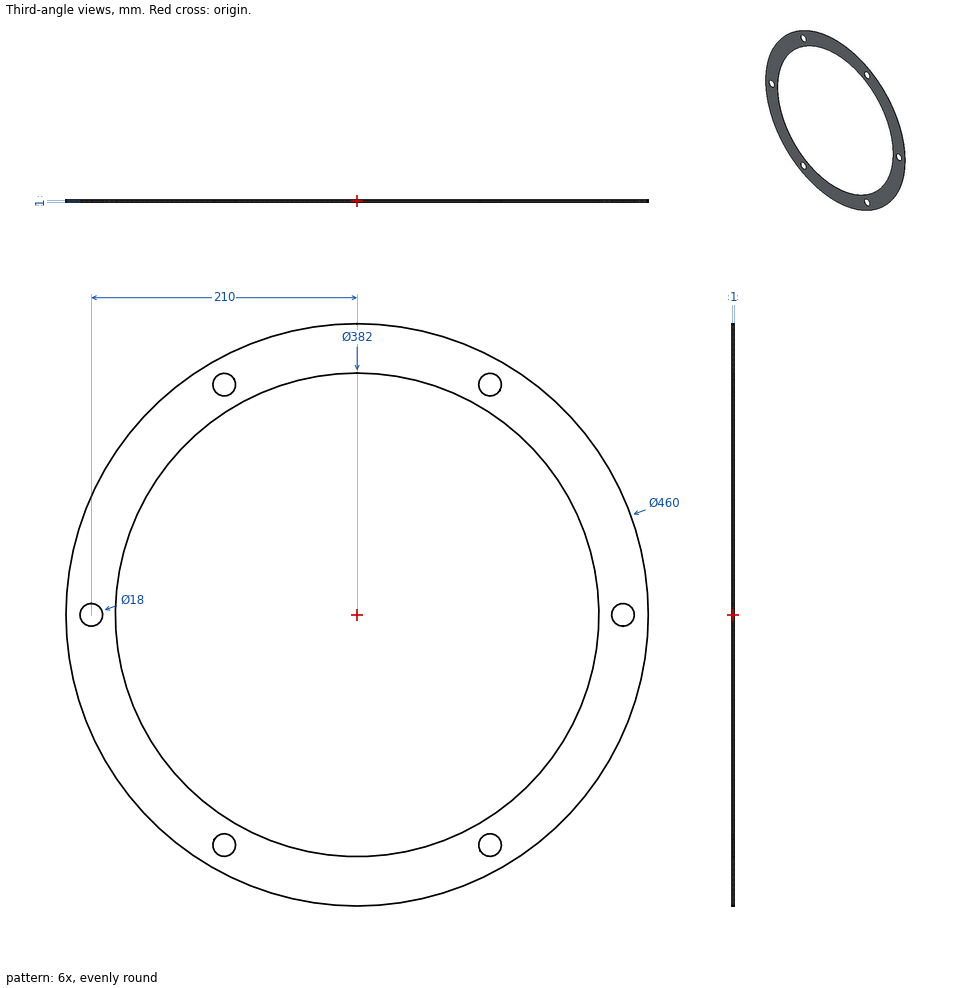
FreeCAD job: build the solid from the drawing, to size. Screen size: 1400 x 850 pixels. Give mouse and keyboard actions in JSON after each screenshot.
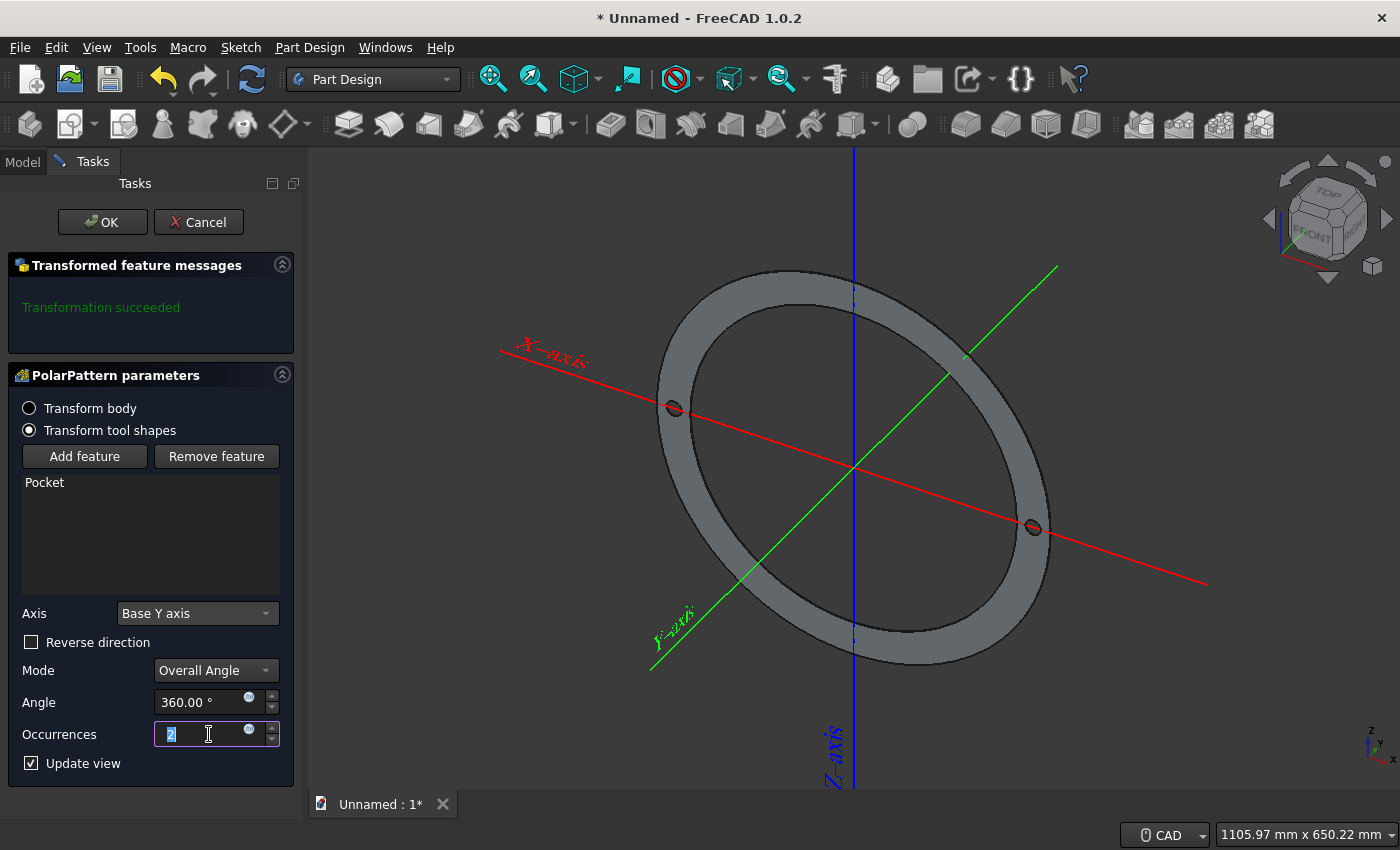
{"action": "type", "text": "6"}
{"action": "key", "text": "Tab"}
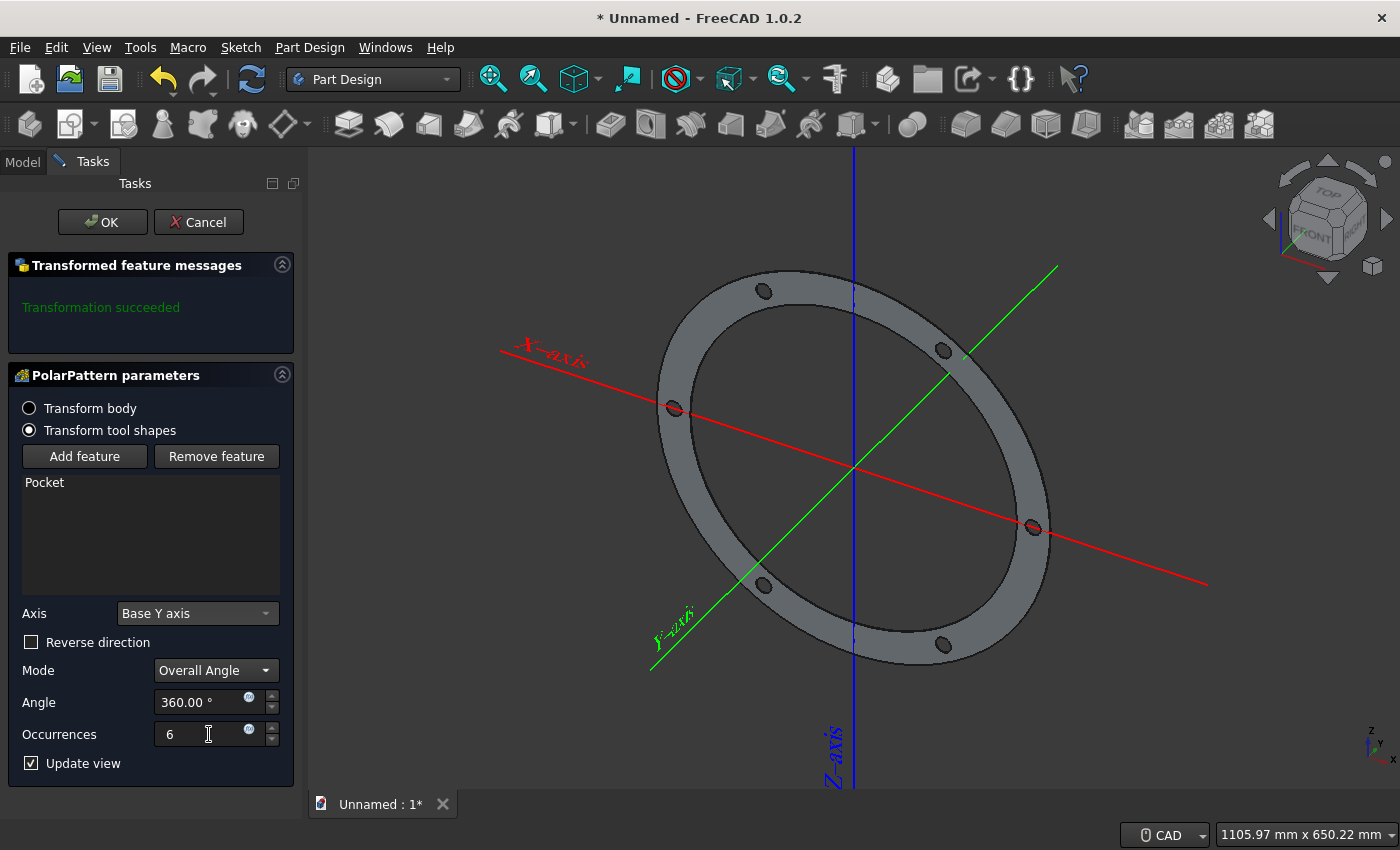
{"action": "left_click", "coordinate": [103, 222]}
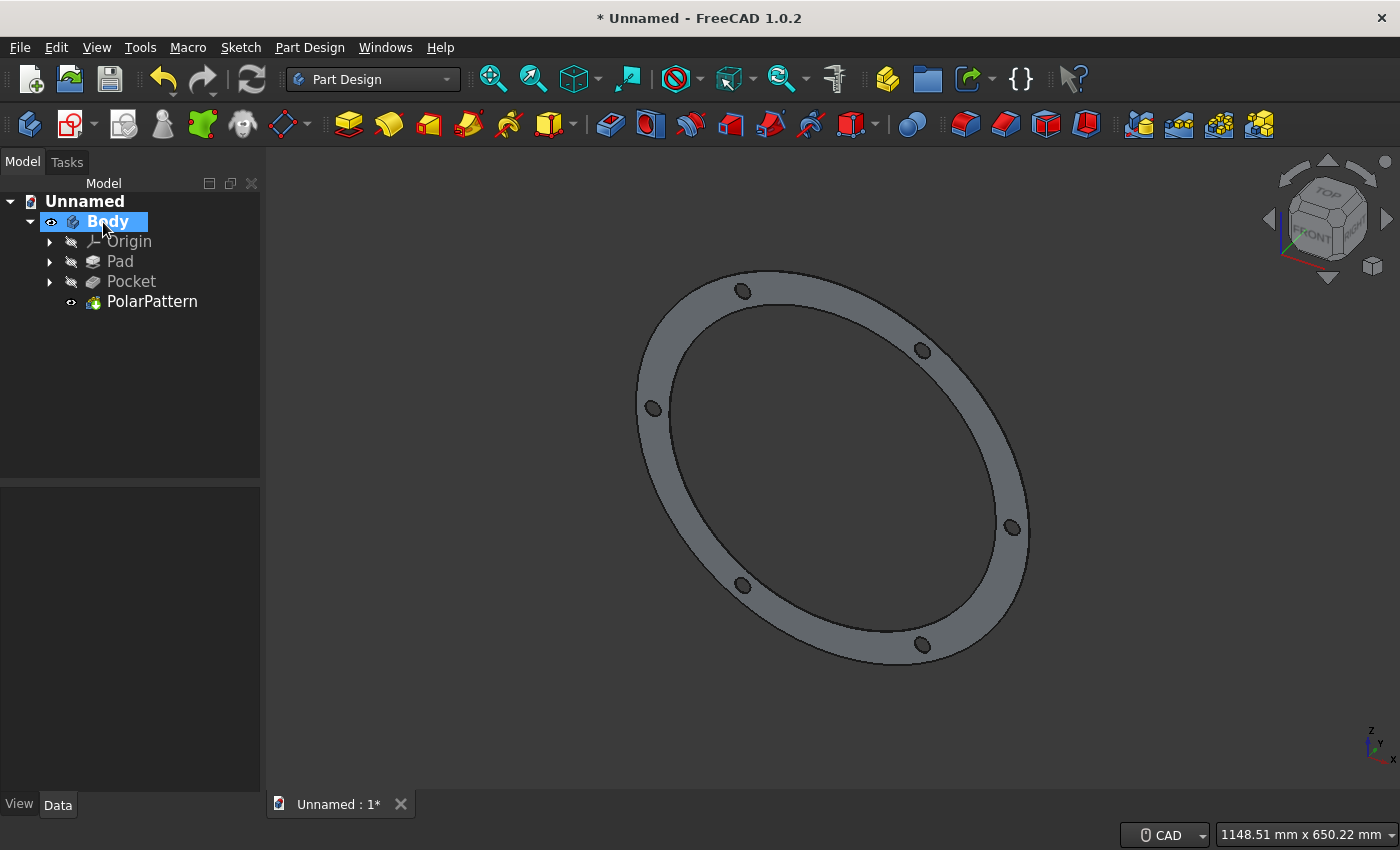
{"action": "key", "text": "0"}